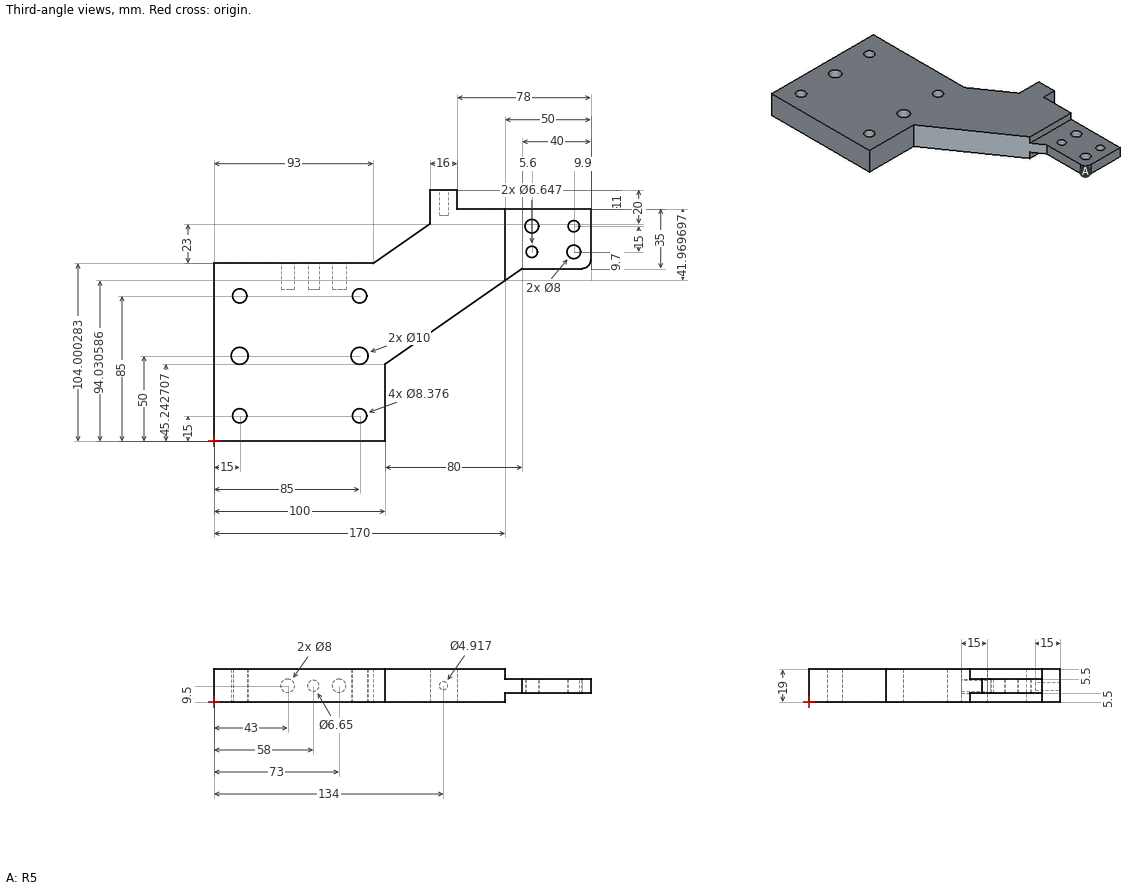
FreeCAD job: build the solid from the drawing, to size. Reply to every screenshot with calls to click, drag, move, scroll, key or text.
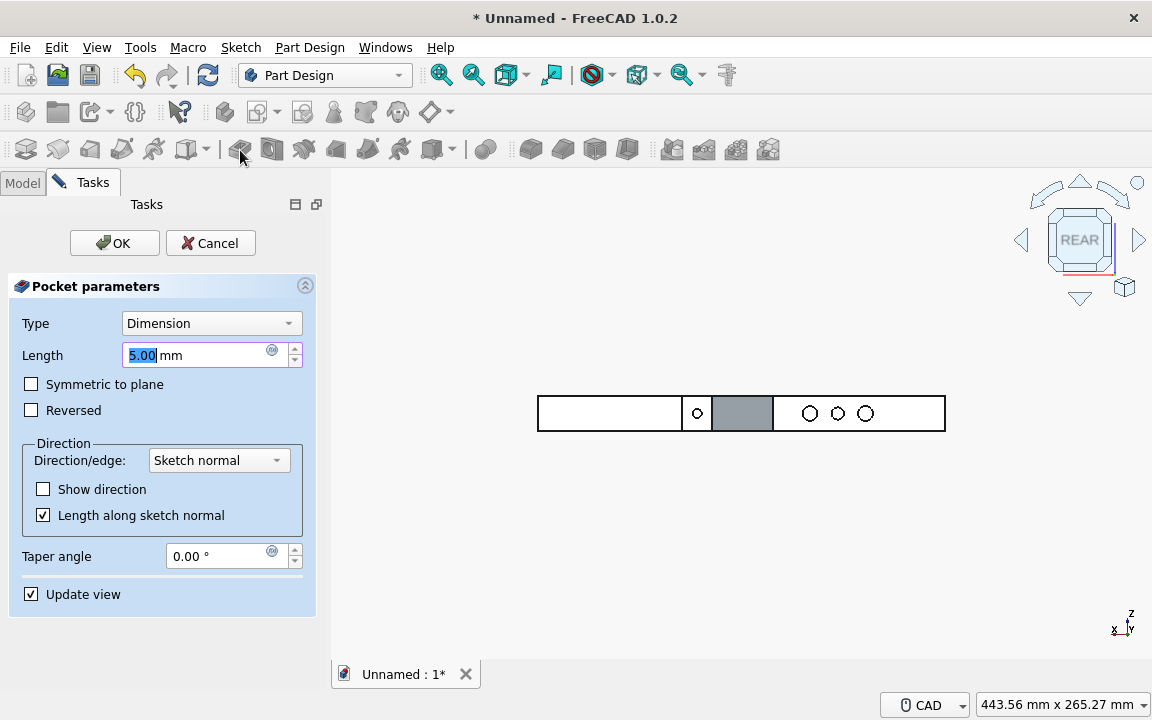
text(15)
key(Tab)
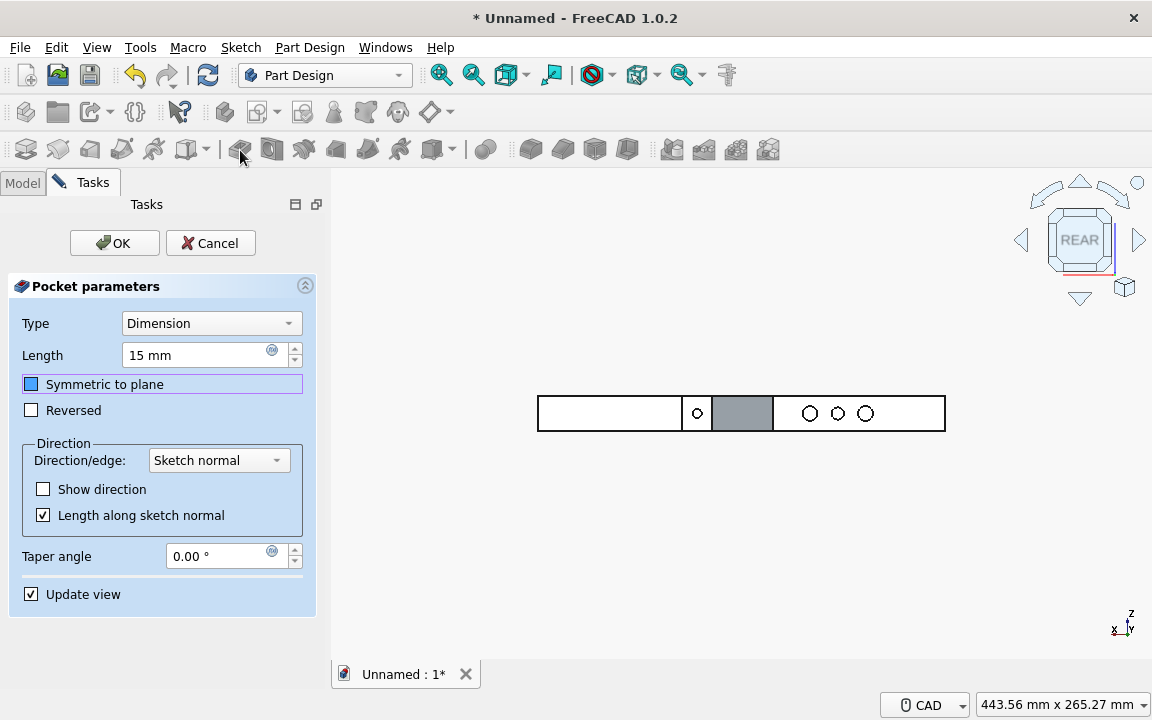
click(115, 243)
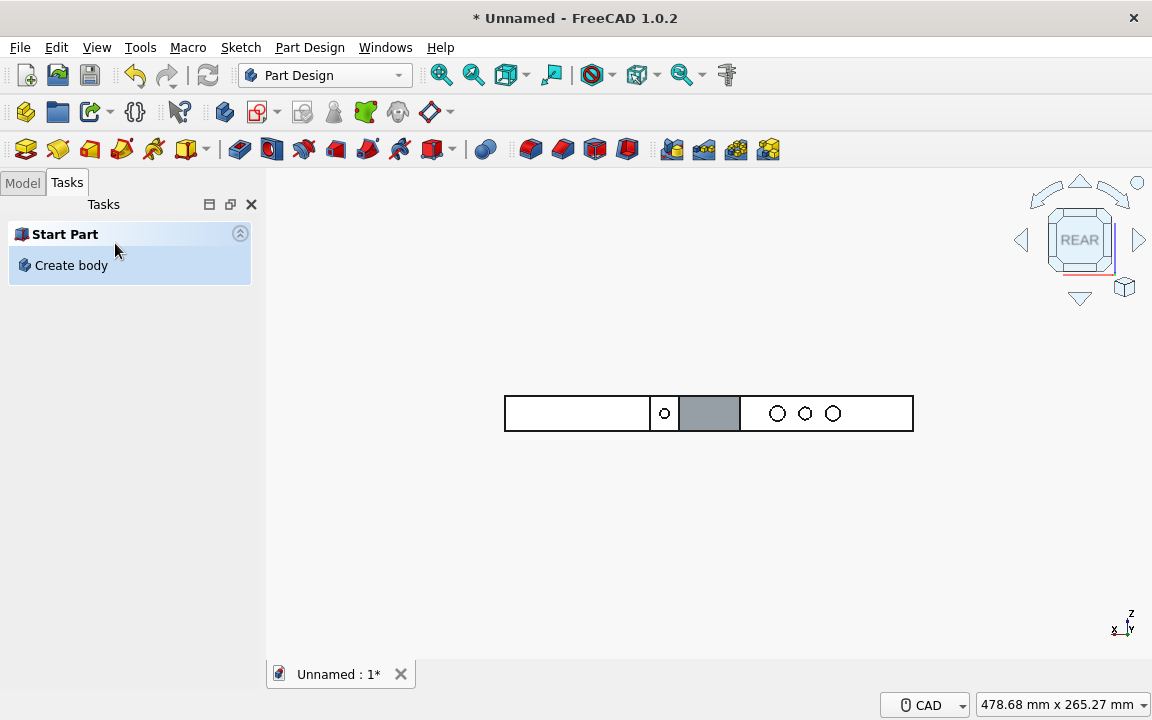
key(0)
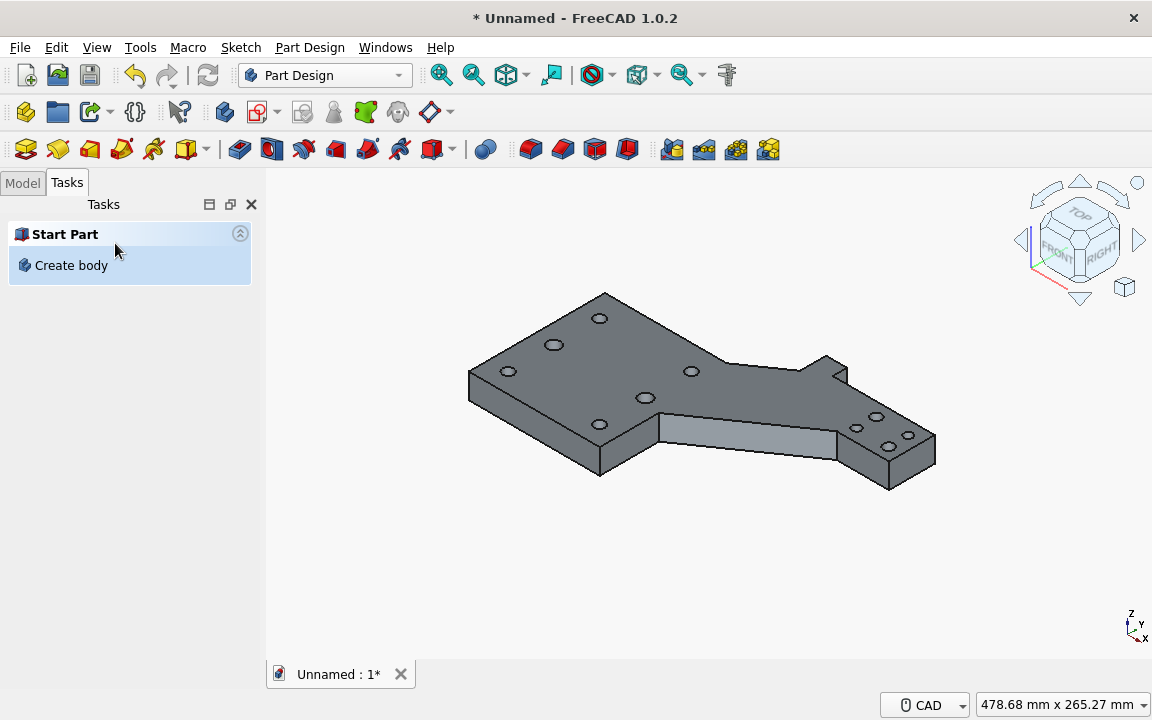
click(572, 382)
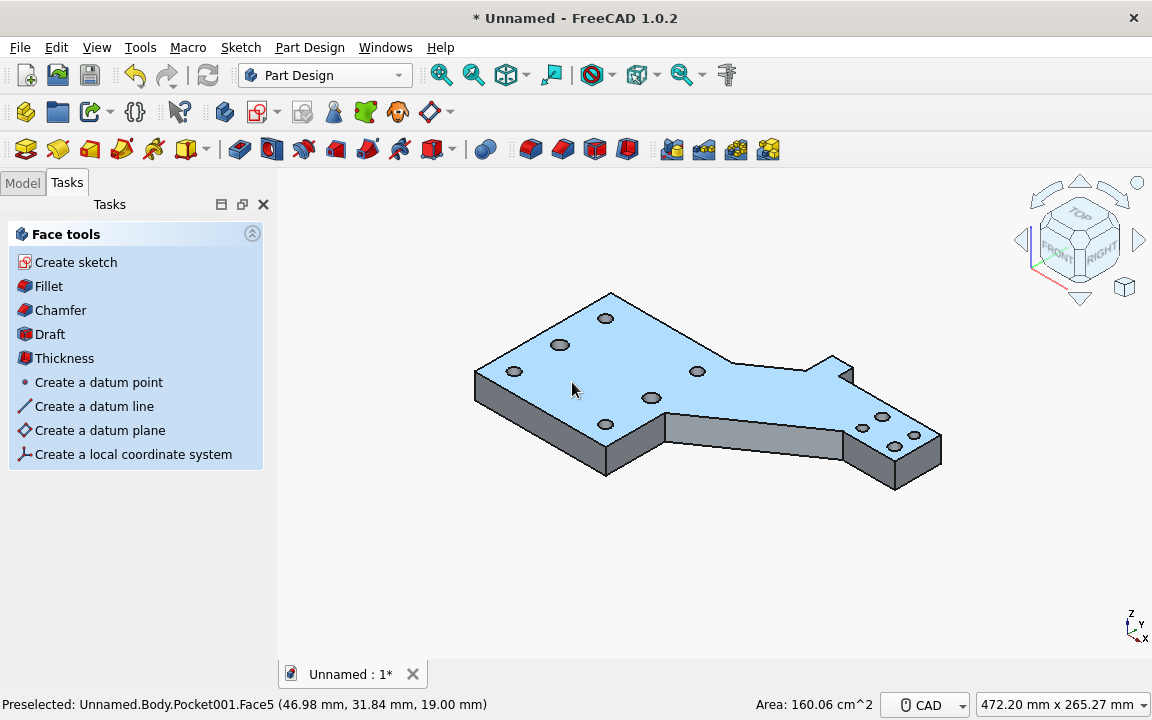
click(258, 112)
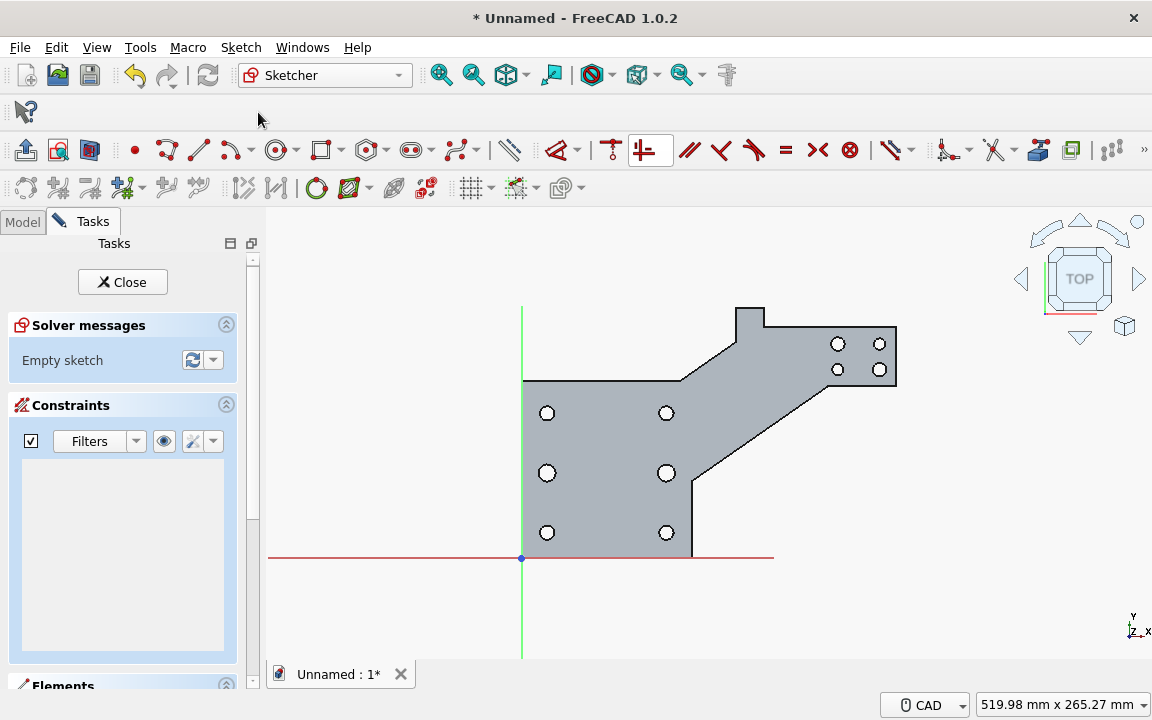
scroll(924, 339, up, 7)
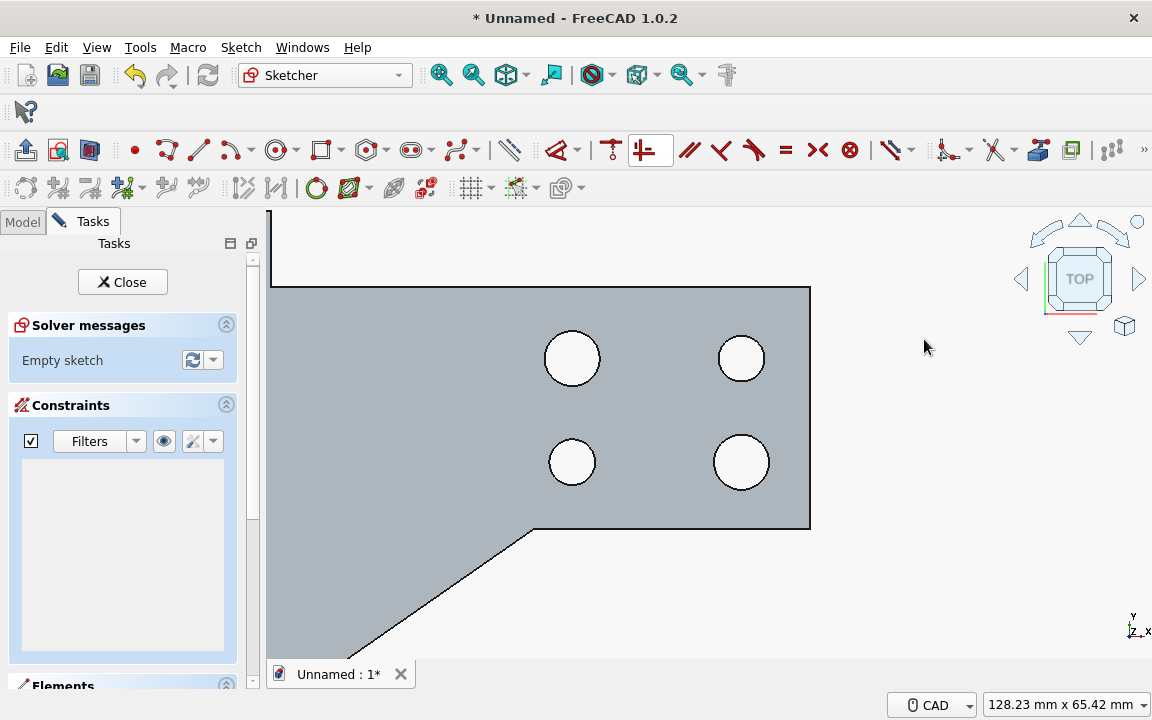
click(322, 150)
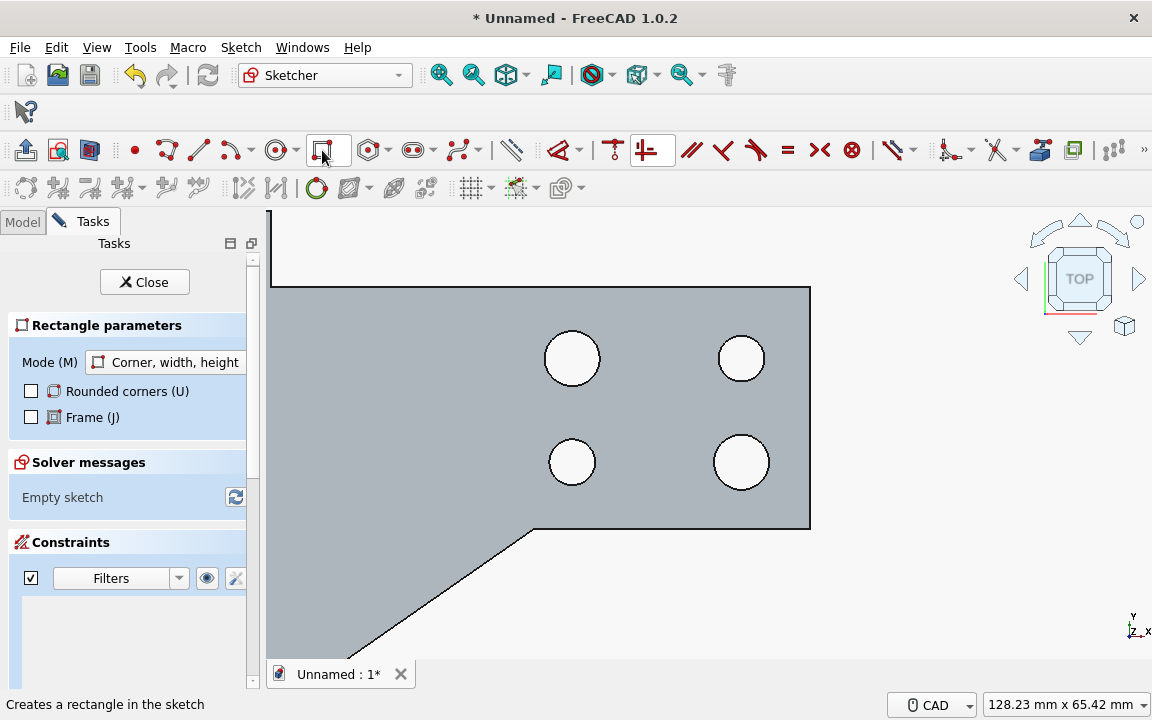
click(464, 287)
click(810, 577)
key(Escape)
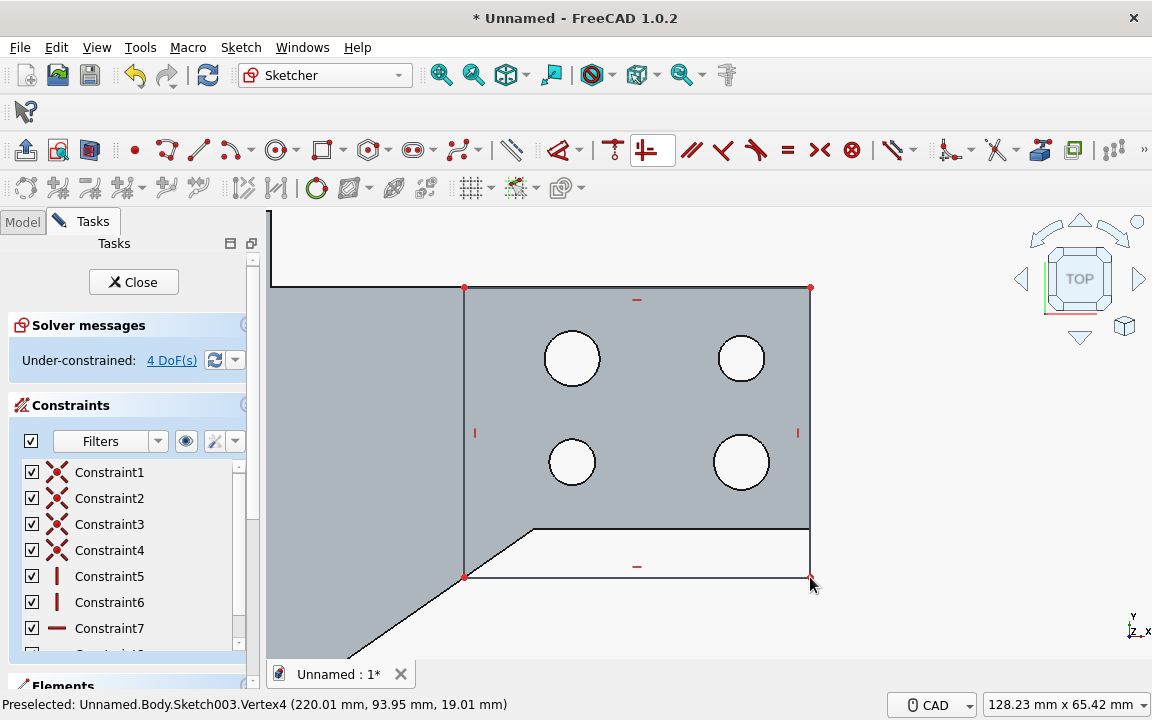
click(558, 150)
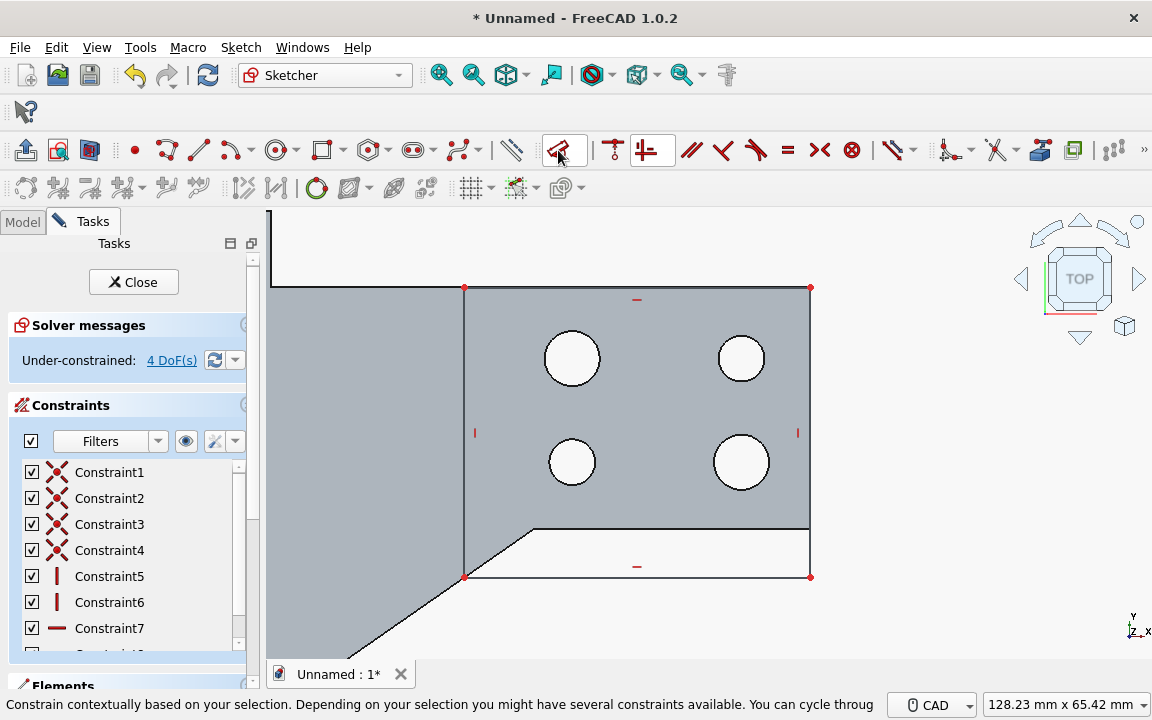
click(568, 578)
click(637, 612)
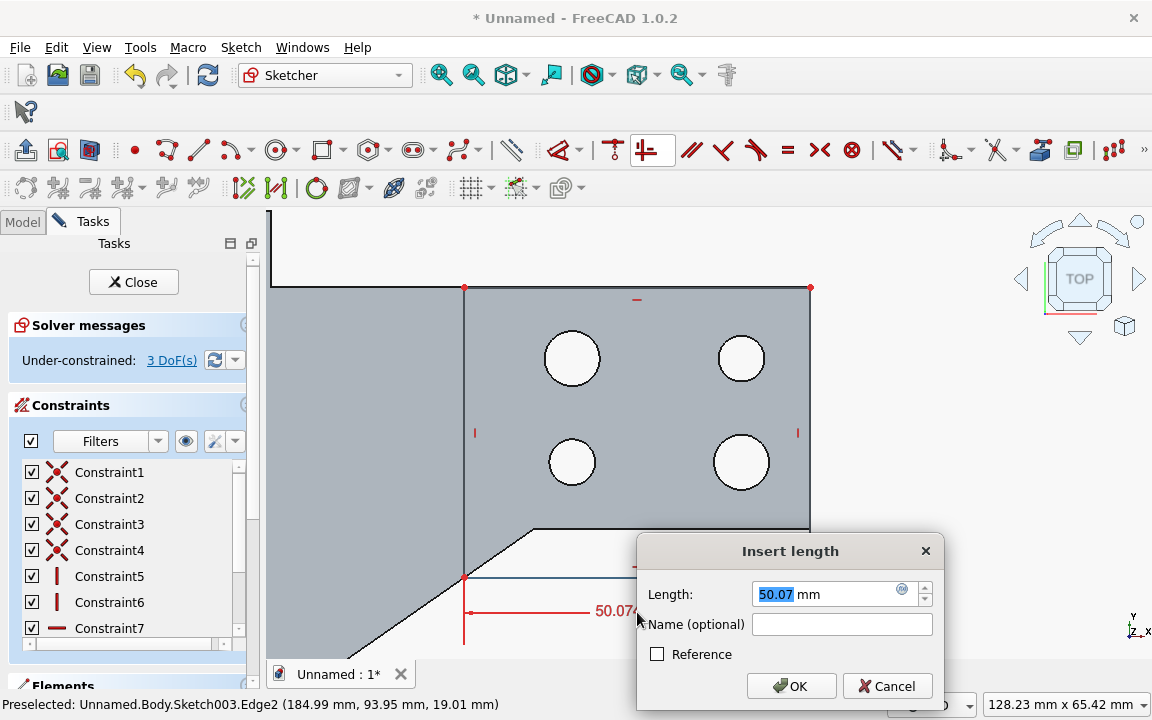
text(50)
key(Return)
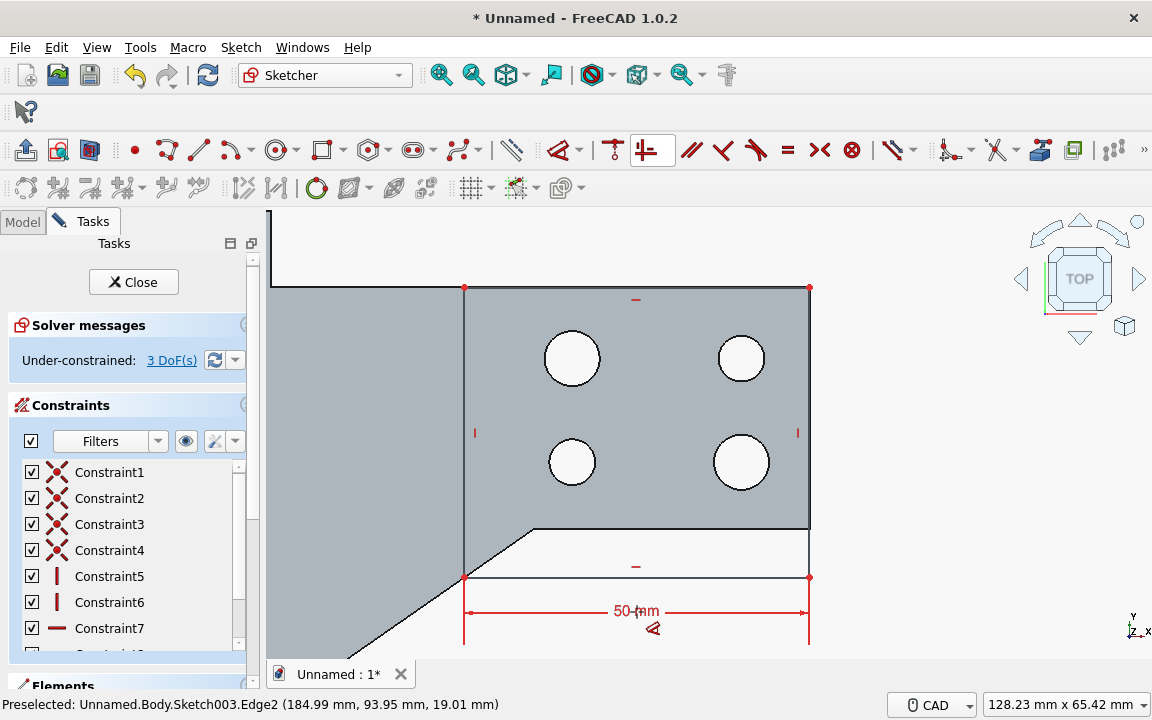
click(464, 288)
click(379, 254)